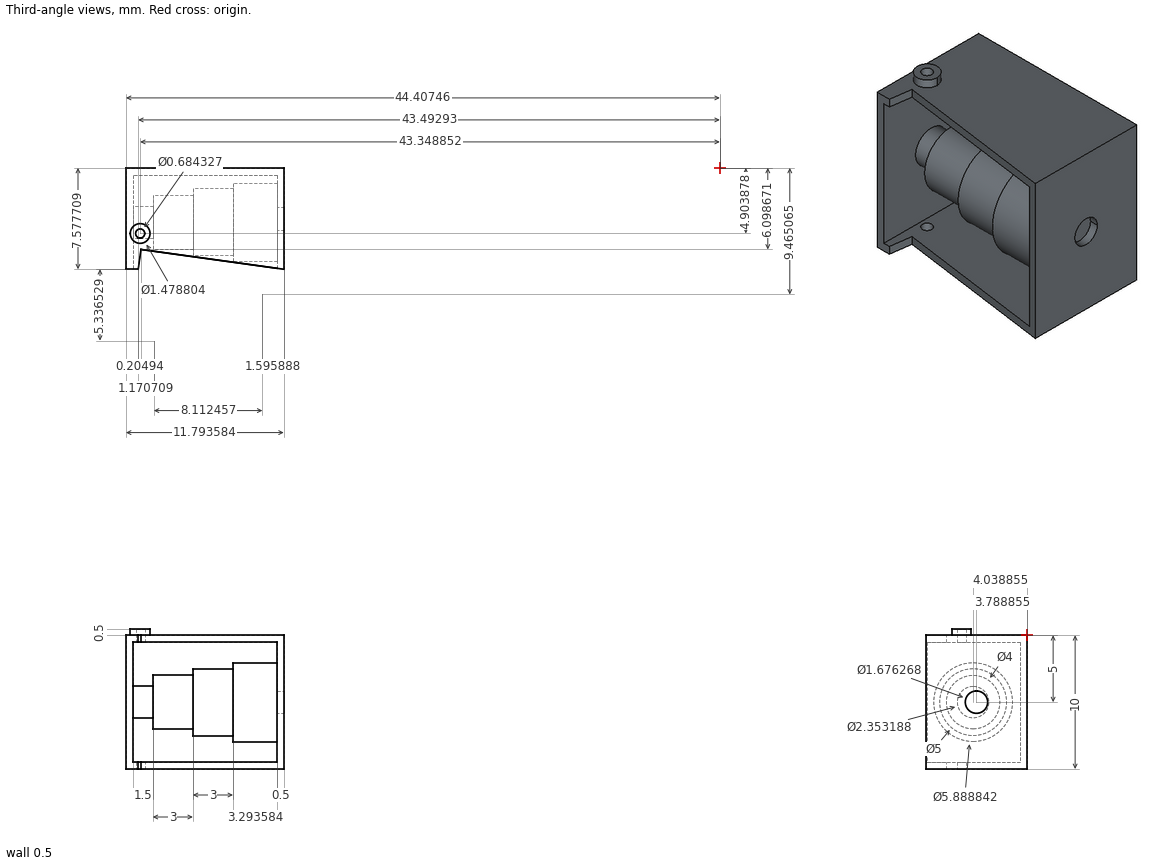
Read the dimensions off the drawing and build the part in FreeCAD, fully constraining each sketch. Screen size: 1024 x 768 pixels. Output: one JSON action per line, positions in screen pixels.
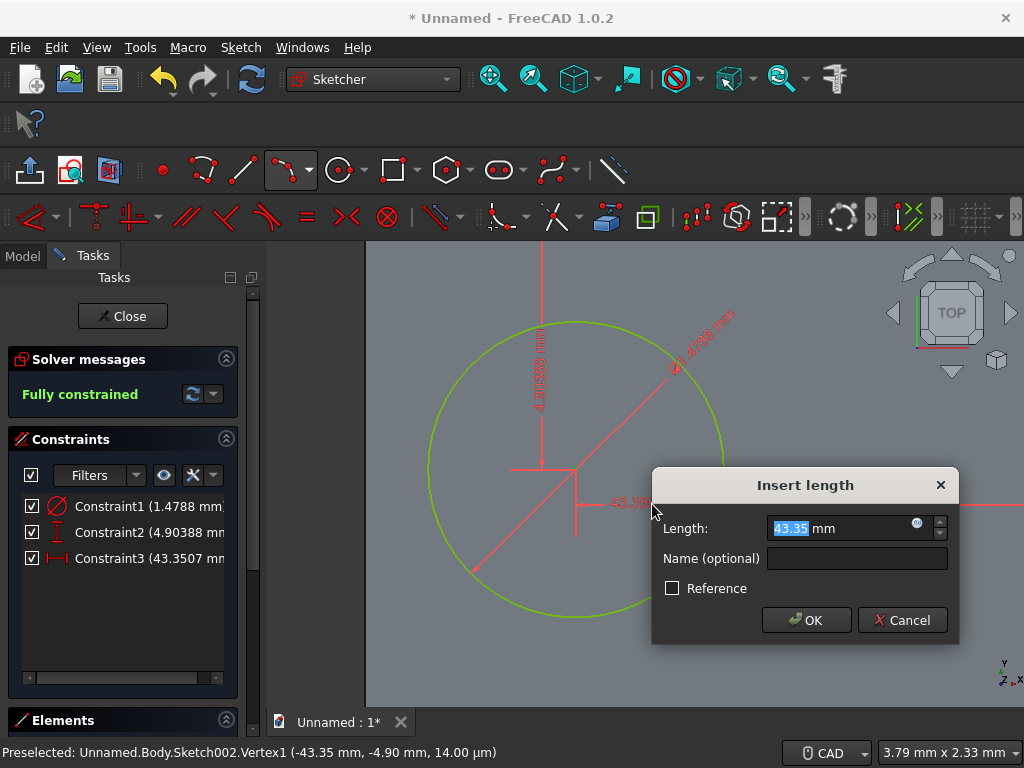
{"action": "type", "text": "43.348852"}
{"action": "key", "text": "Return"}
{"action": "key", "text": "Escape"}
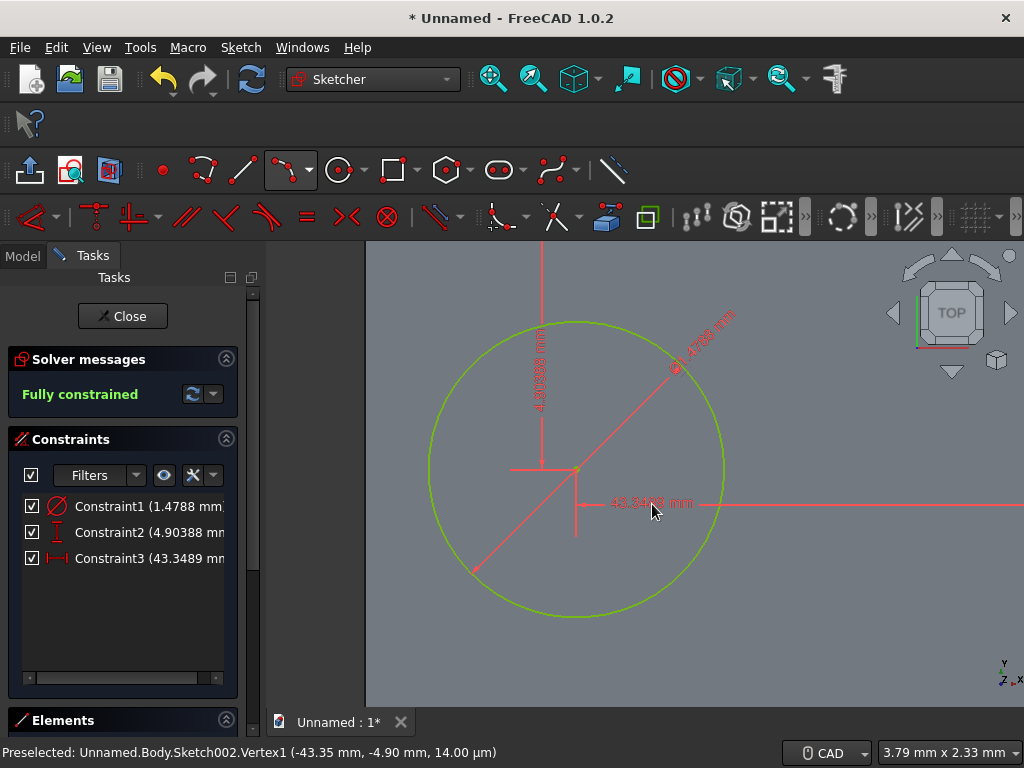
{"action": "left_click", "coordinate": [123, 316]}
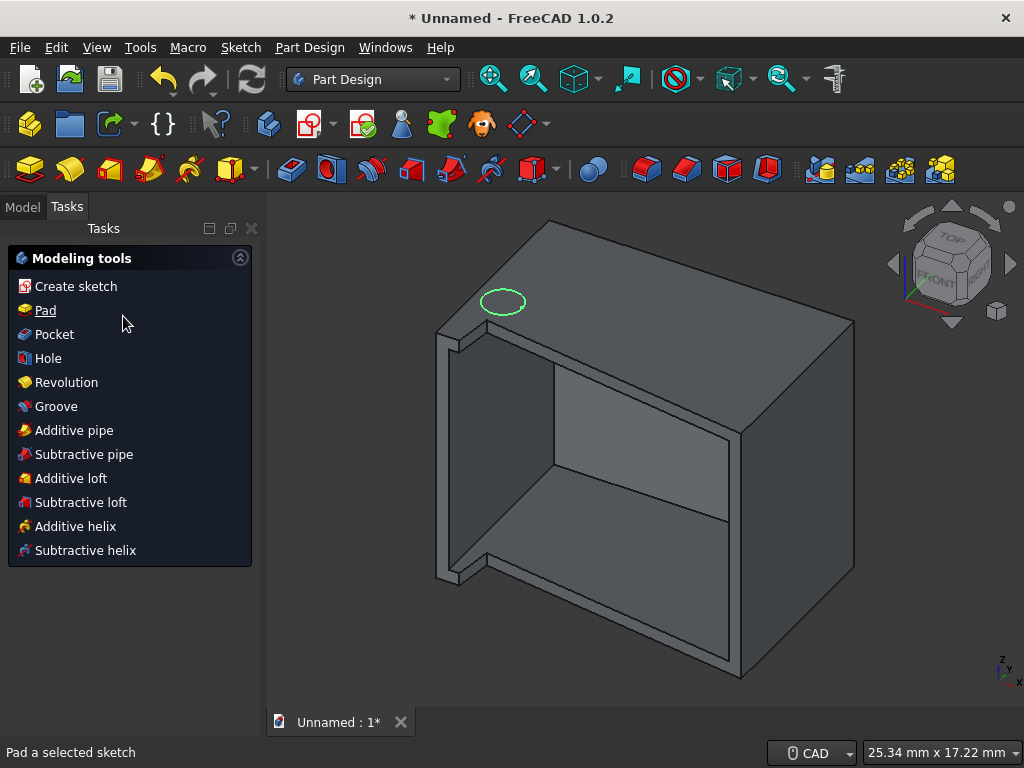
{"action": "left_click", "coordinate": [30, 170]}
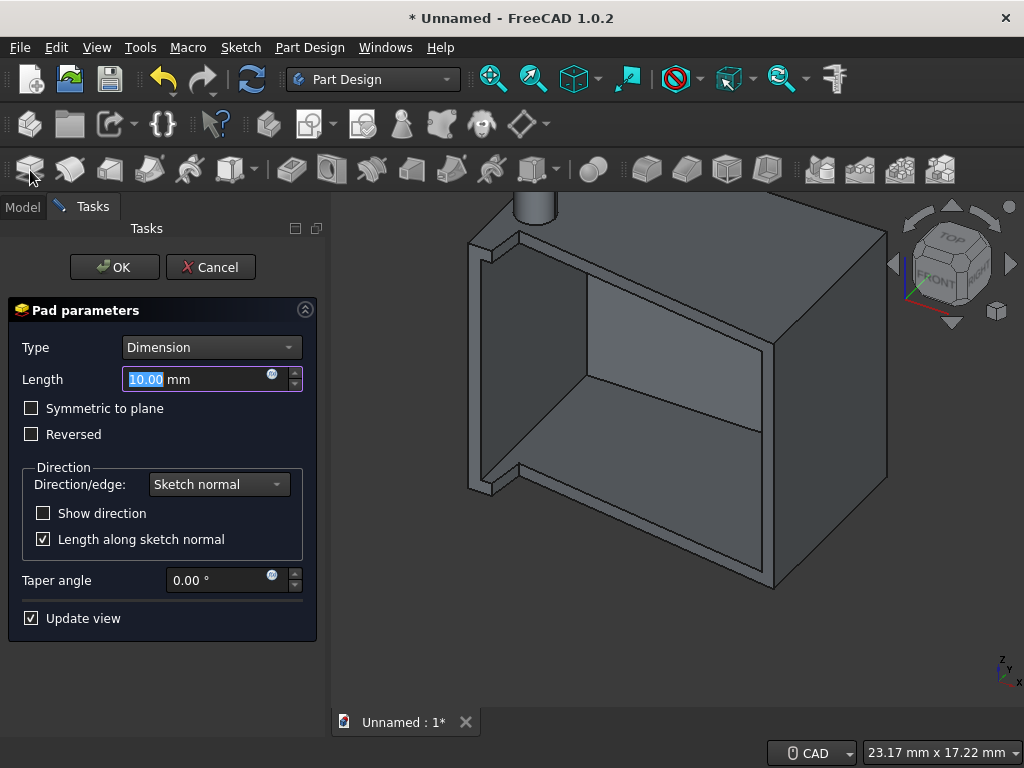
{"action": "type", "text": "0.5"}
{"action": "key", "text": "Tab"}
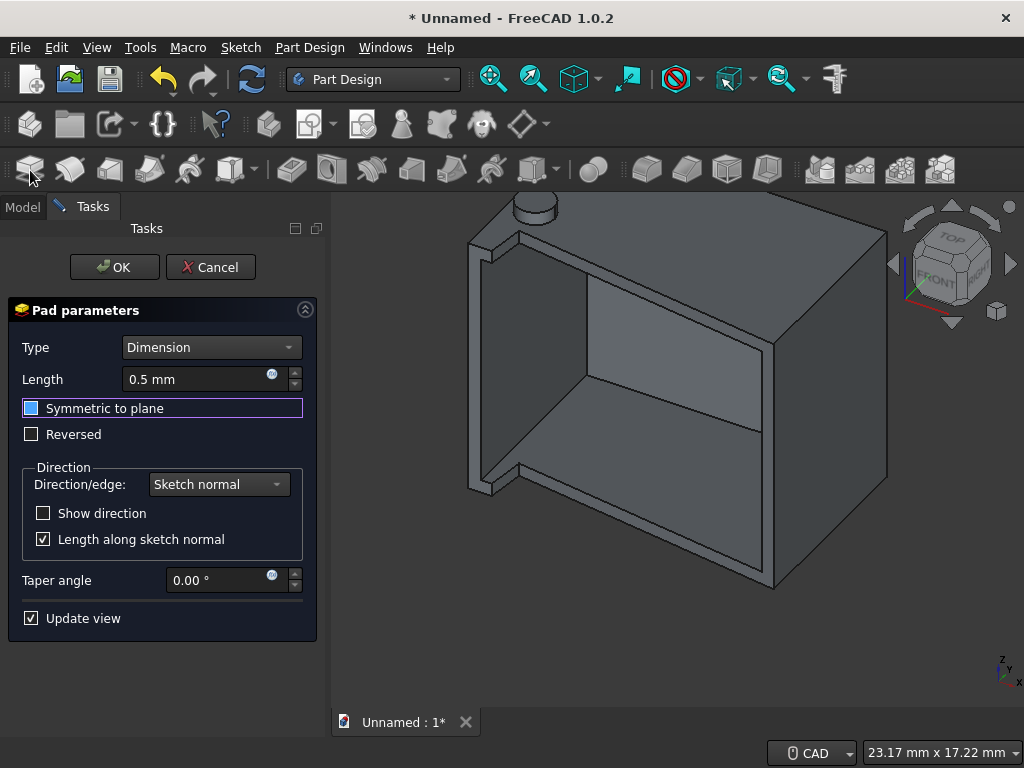
{"action": "left_click", "coordinate": [115, 267]}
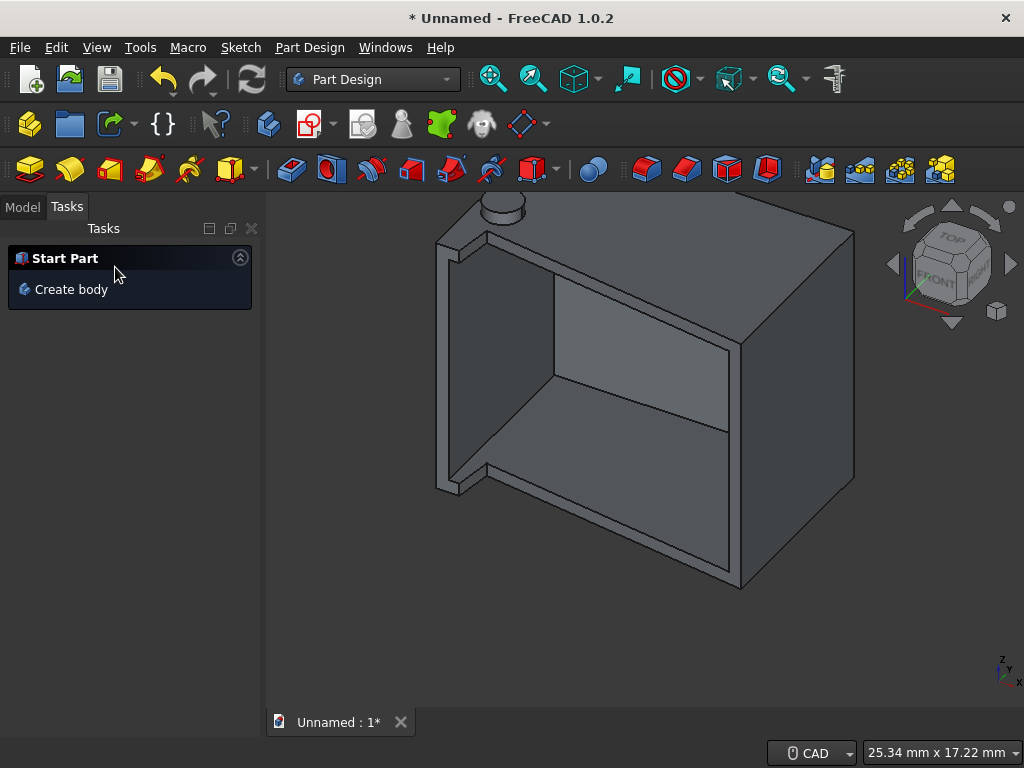
{"action": "left_click", "coordinate": [494, 80]}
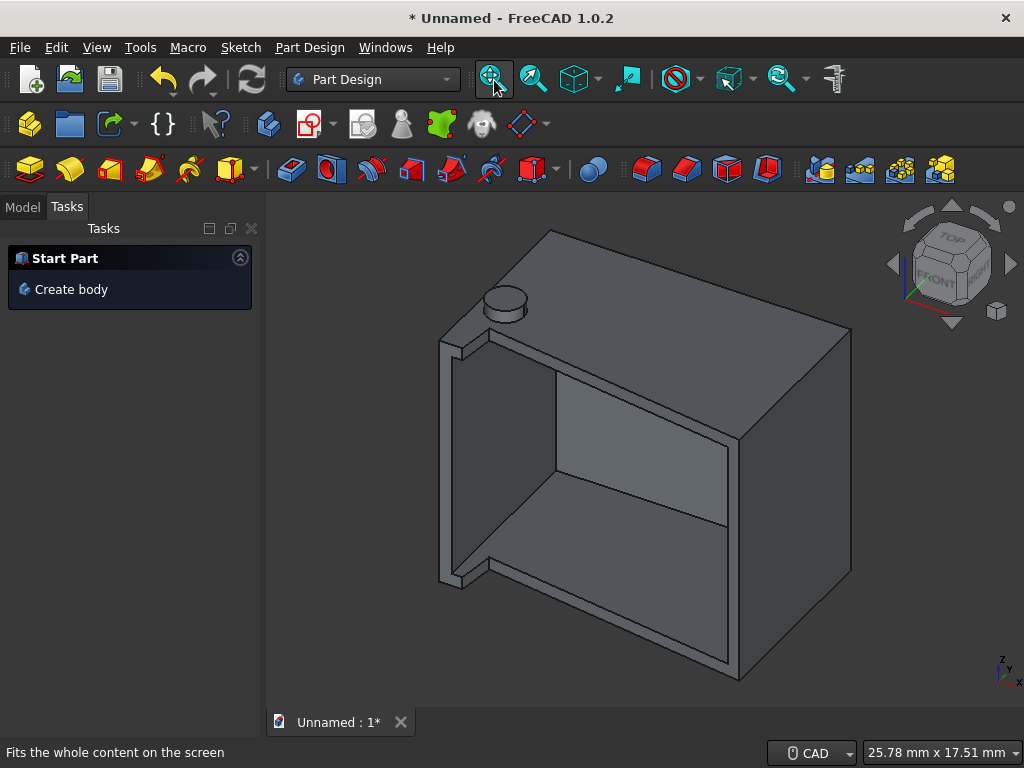
{"action": "left_click", "coordinate": [505, 298]}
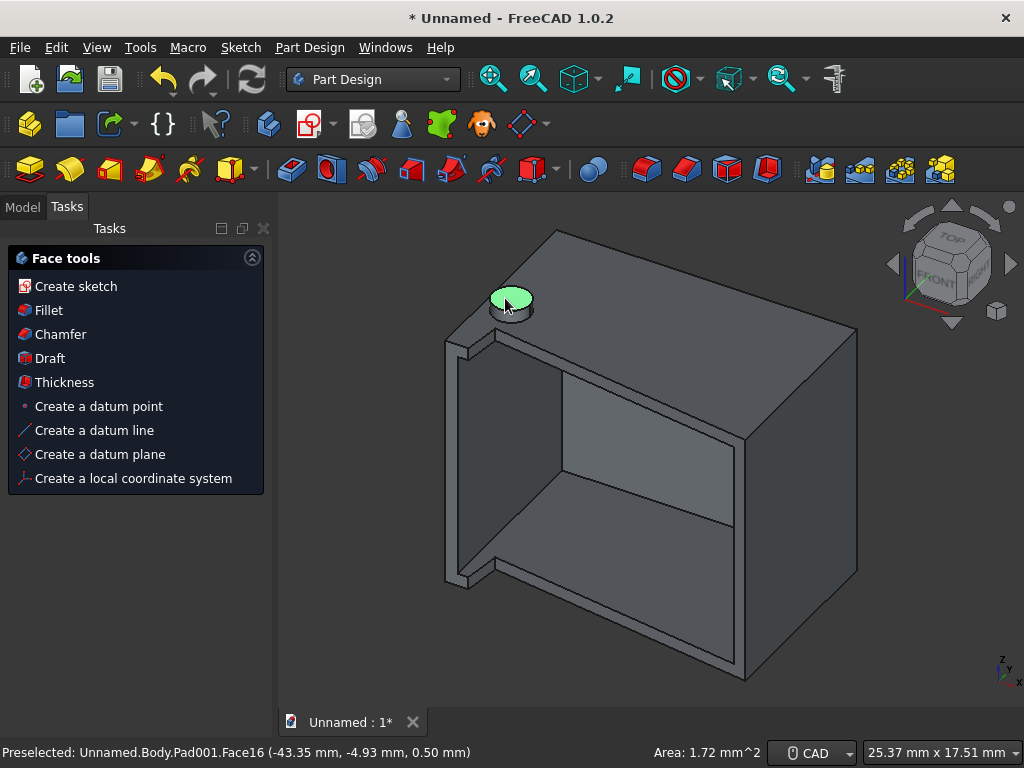
{"action": "left_click", "coordinate": [310, 124]}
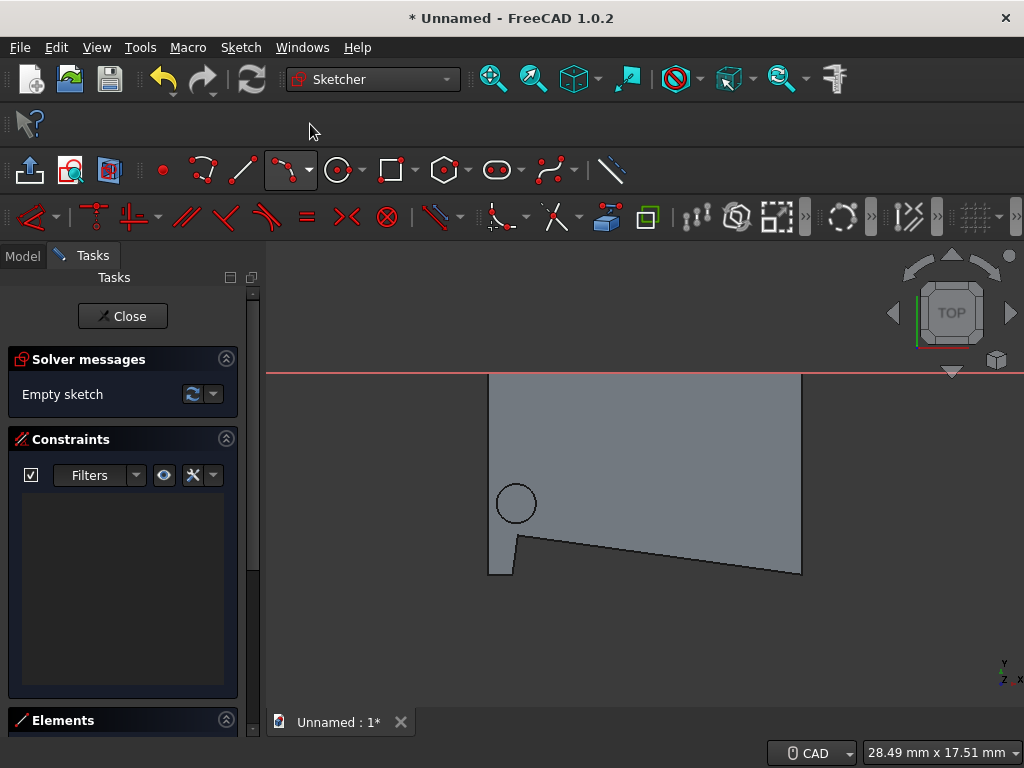
{"action": "scroll", "coordinate": [512, 506], "scroll_direction": "up", "scroll_amount": 14}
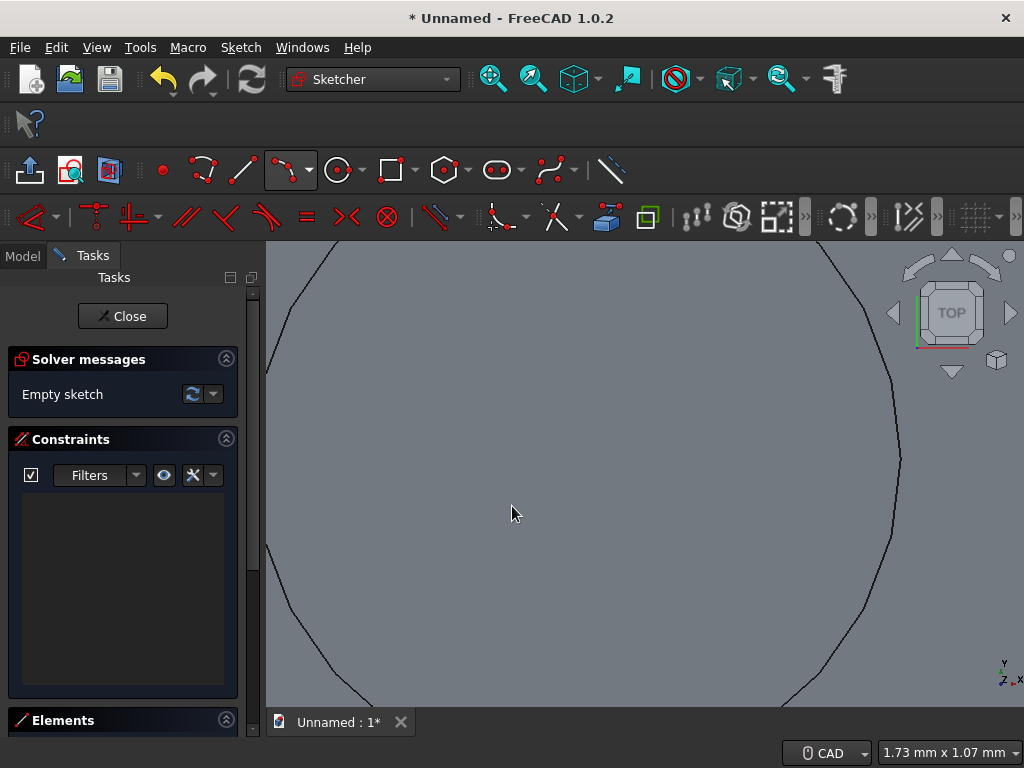
{"action": "left_click", "coordinate": [338, 170]}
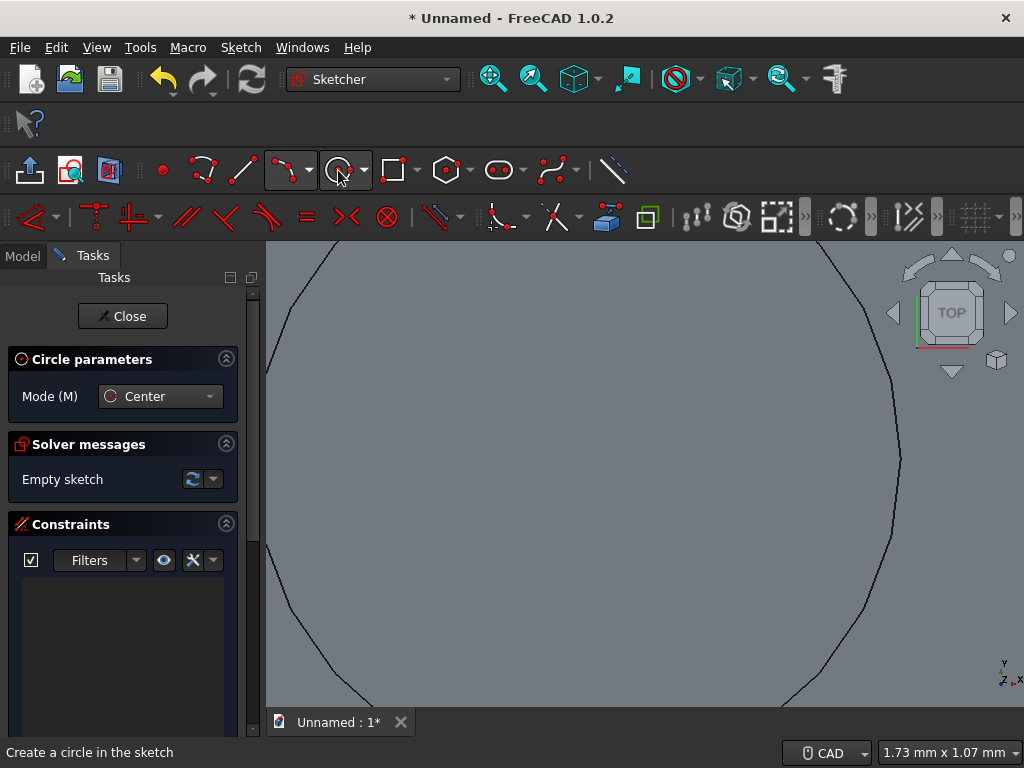
{"action": "left_click", "coordinate": [577, 459]}
{"action": "left_click", "coordinate": [683, 353]}
{"action": "key", "text": "Escape"}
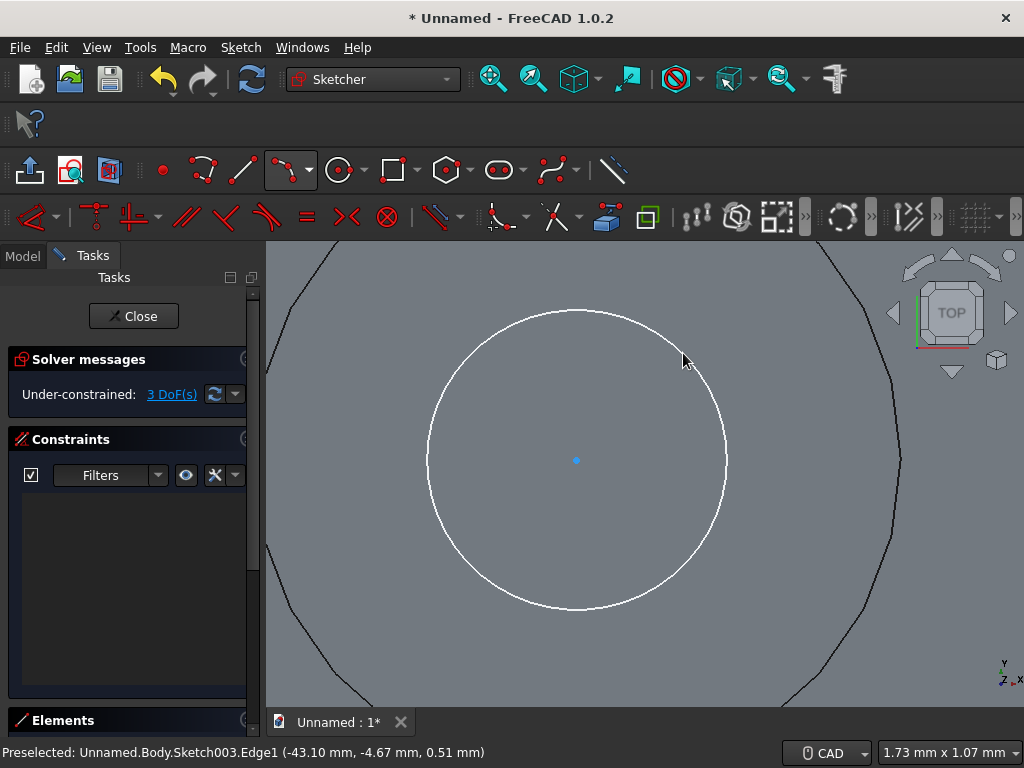
{"action": "left_click", "coordinate": [32, 218]}